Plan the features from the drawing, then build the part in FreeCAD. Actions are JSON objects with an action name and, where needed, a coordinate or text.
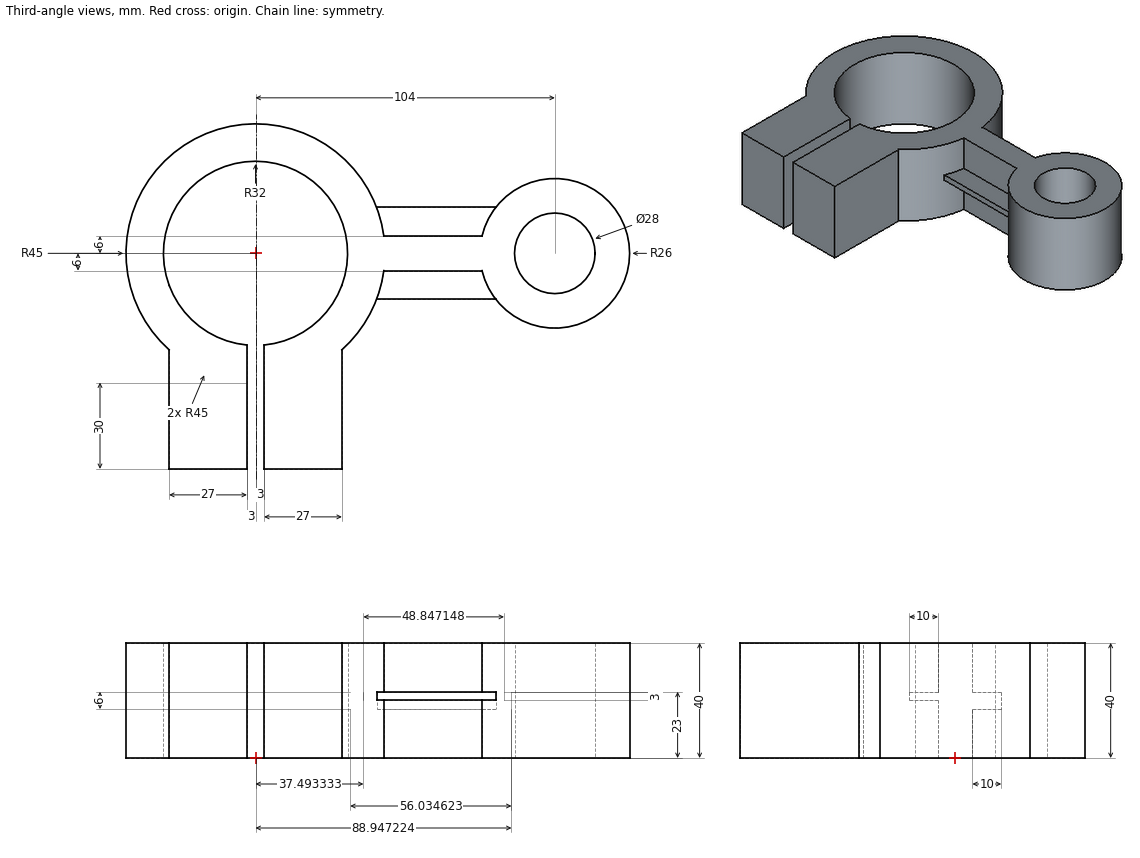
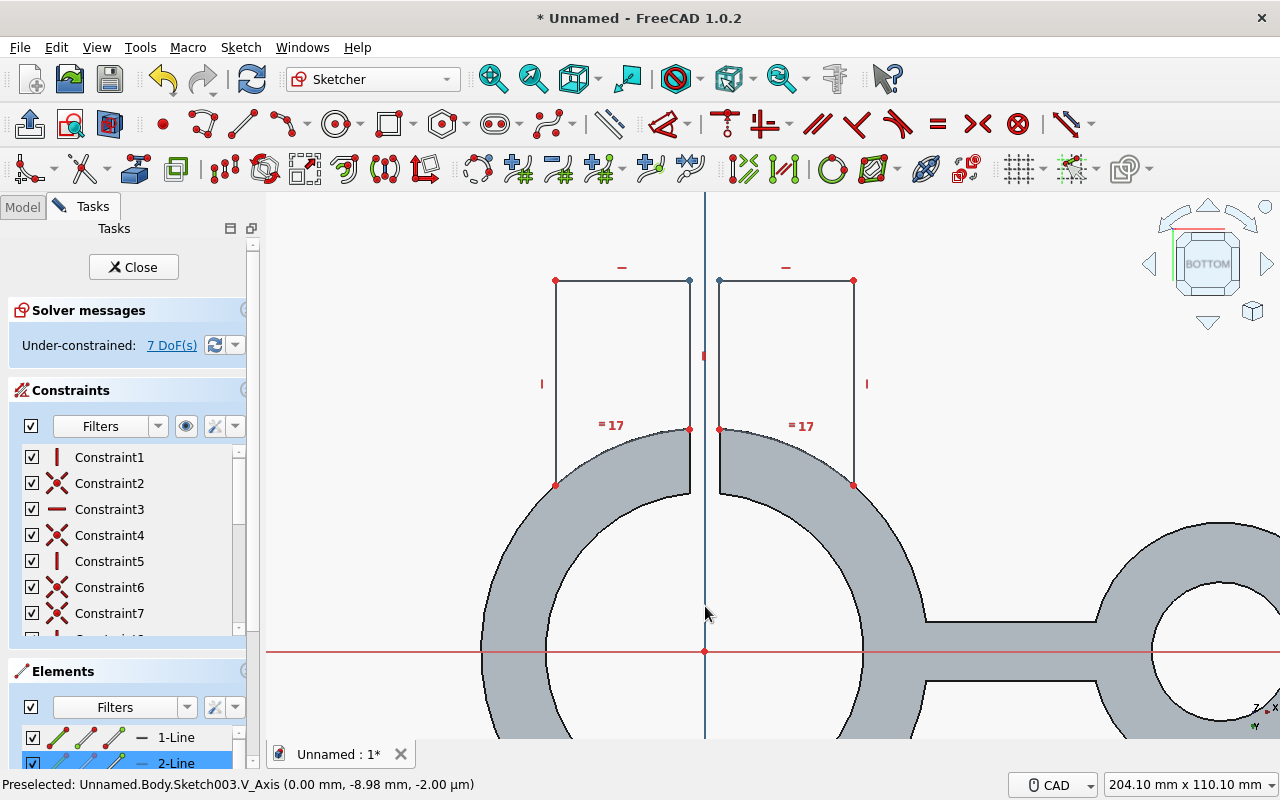
{"action": "left_click", "coordinate": [978, 124]}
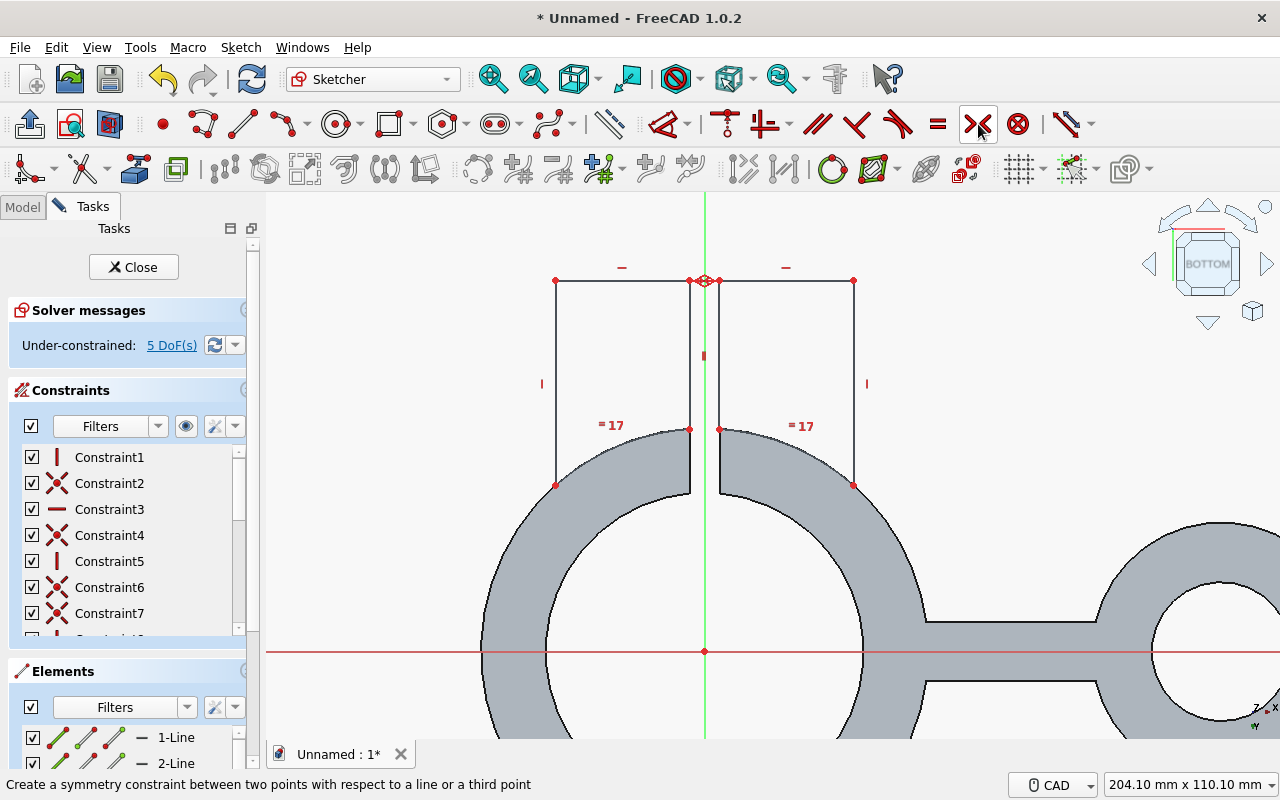
{"action": "left_click", "coordinate": [664, 124]}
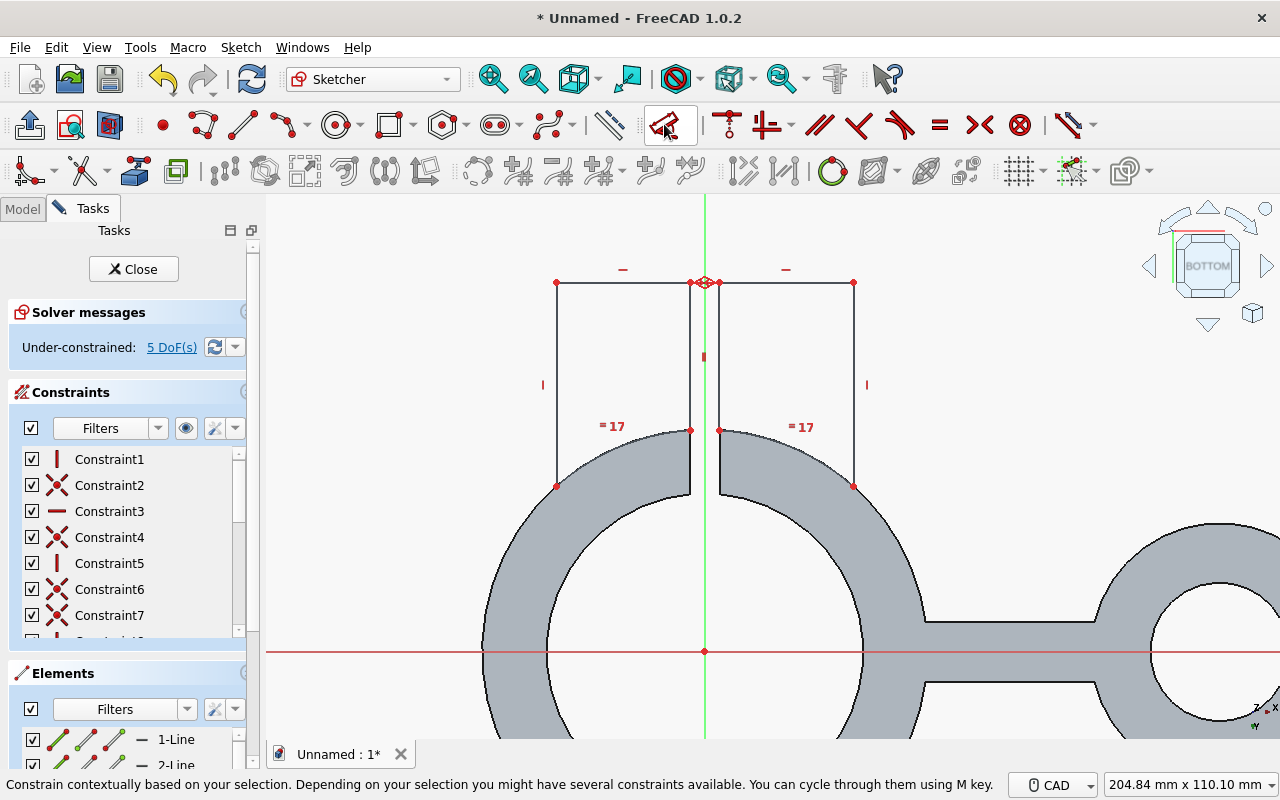
{"action": "left_click", "coordinate": [647, 437]}
{"action": "left_click", "coordinate": [639, 406]}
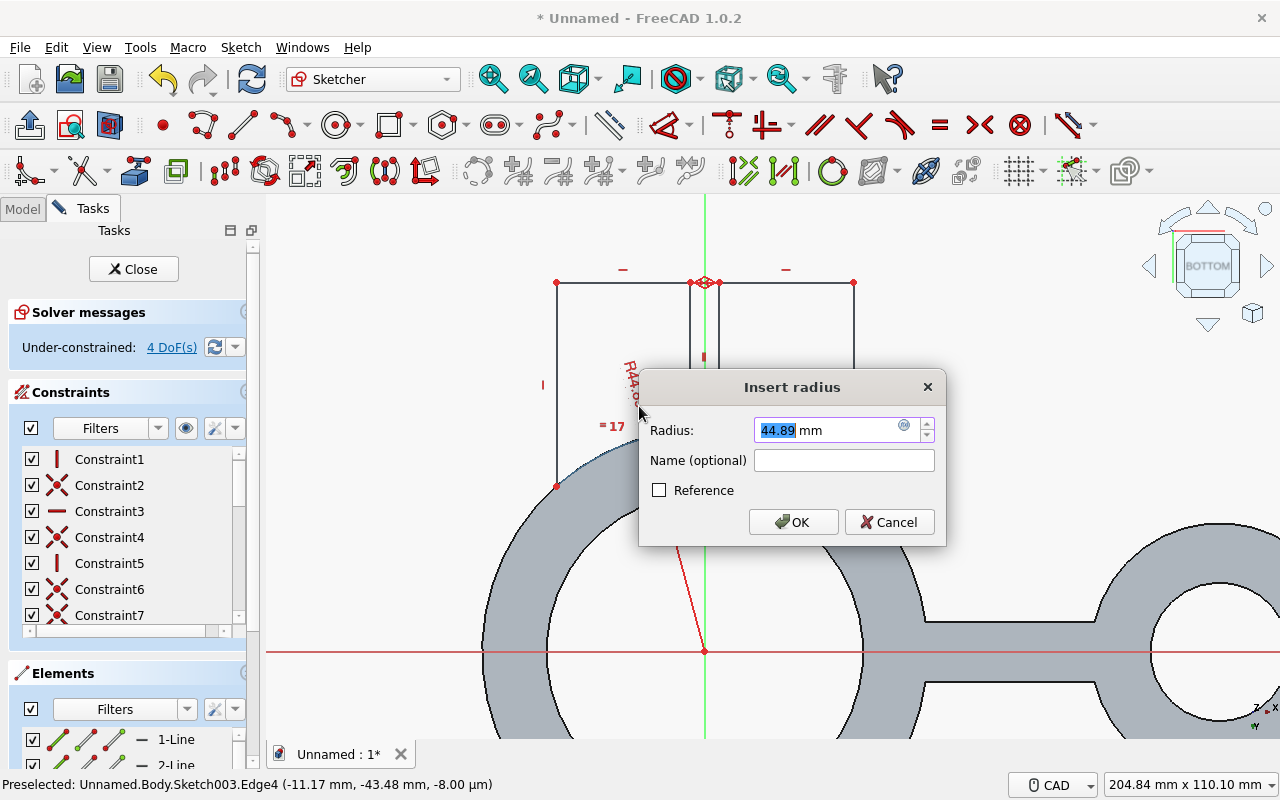
{"action": "type", "text": "45"}
{"action": "key", "text": "Return"}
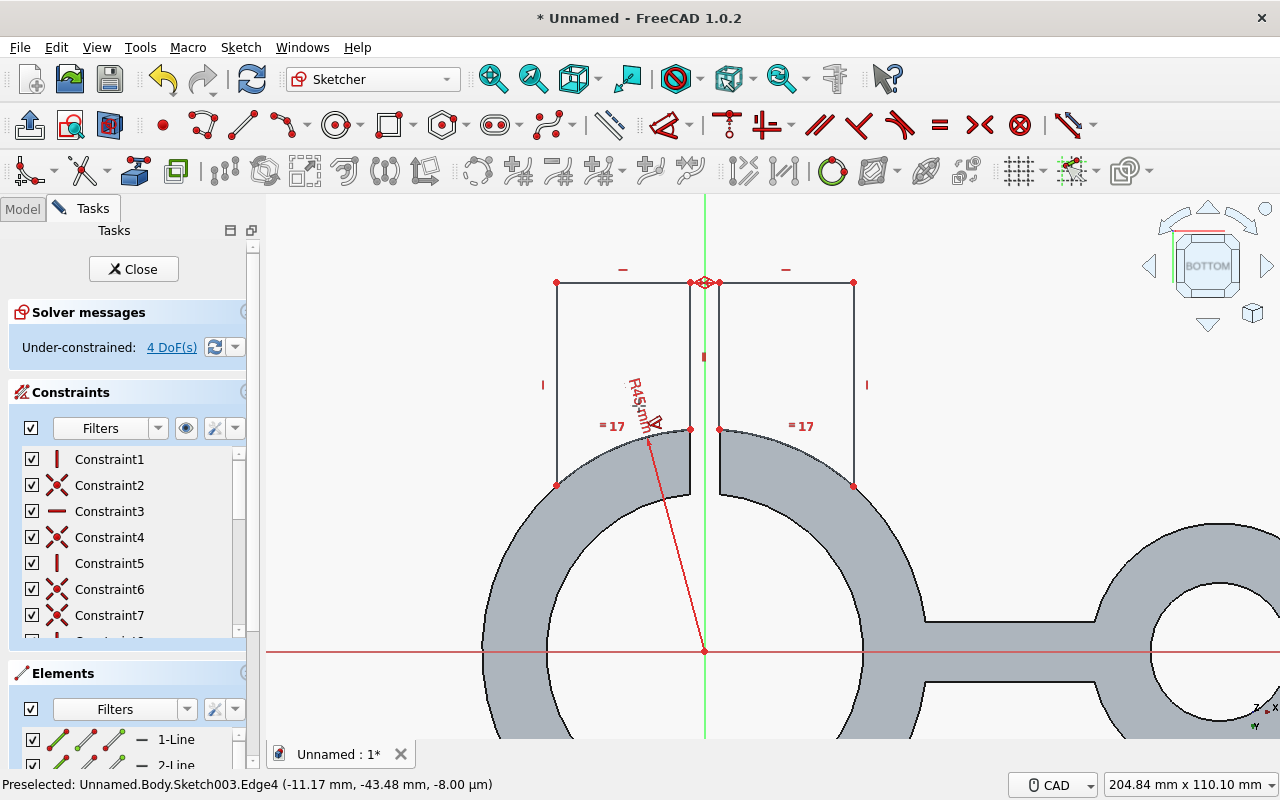
{"action": "left_click", "coordinate": [597, 283]}
{"action": "left_click", "coordinate": [624, 249]}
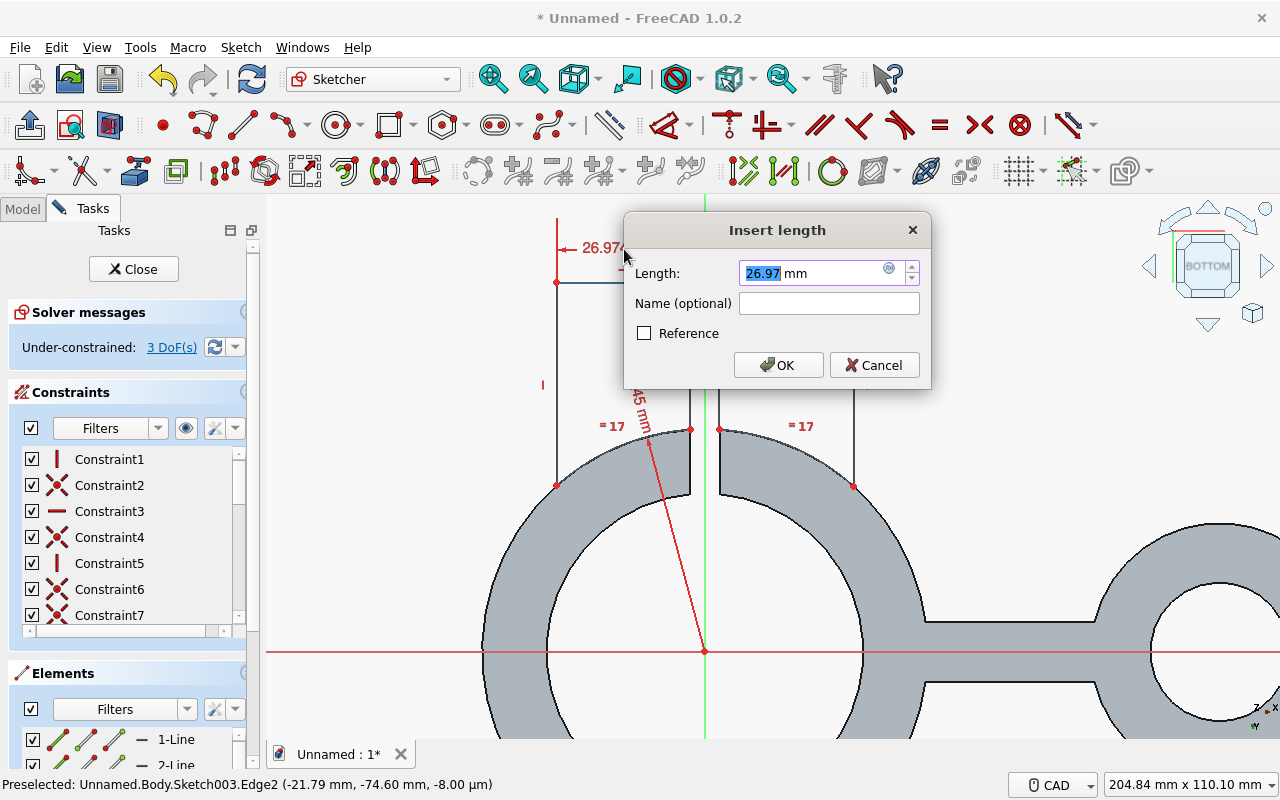
{"action": "type", "text": "27"}
{"action": "key", "text": "Return"}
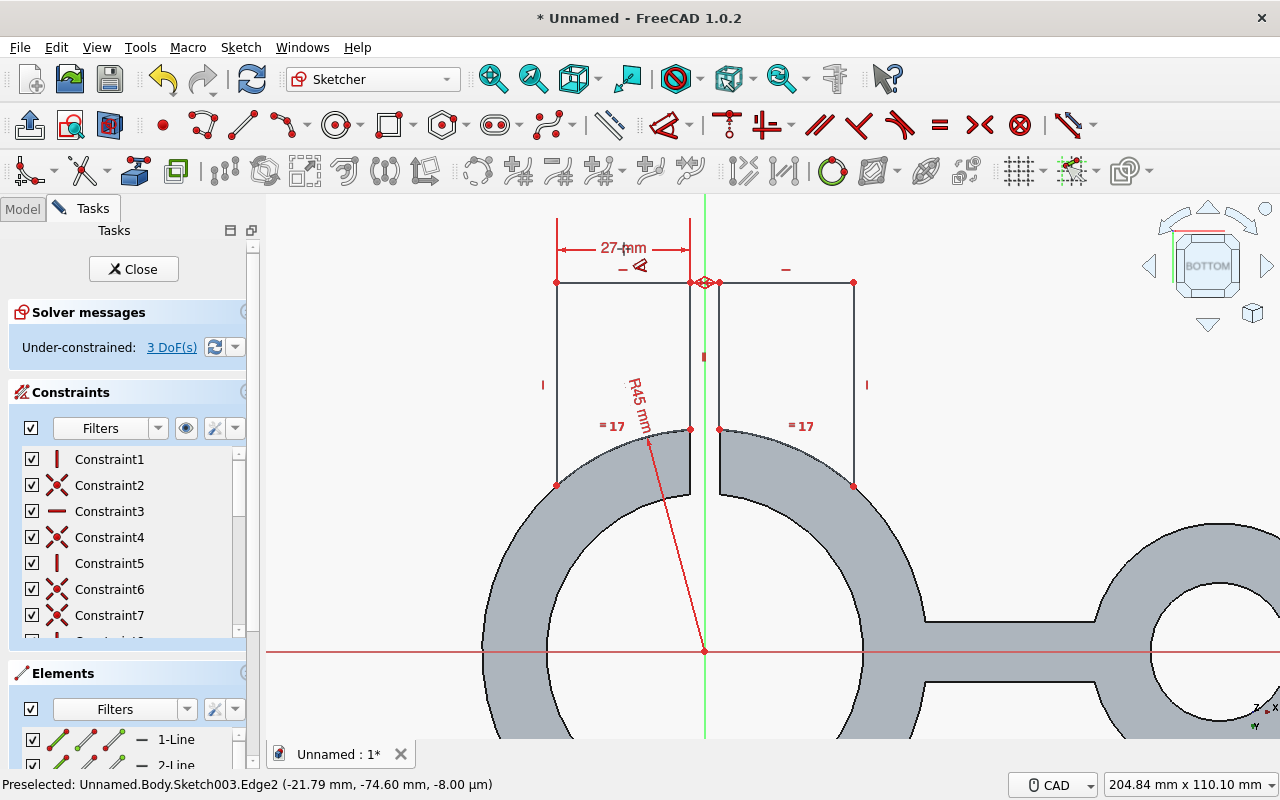
{"action": "left_click", "coordinate": [690, 327]}
{"action": "left_click", "coordinate": [656, 356]}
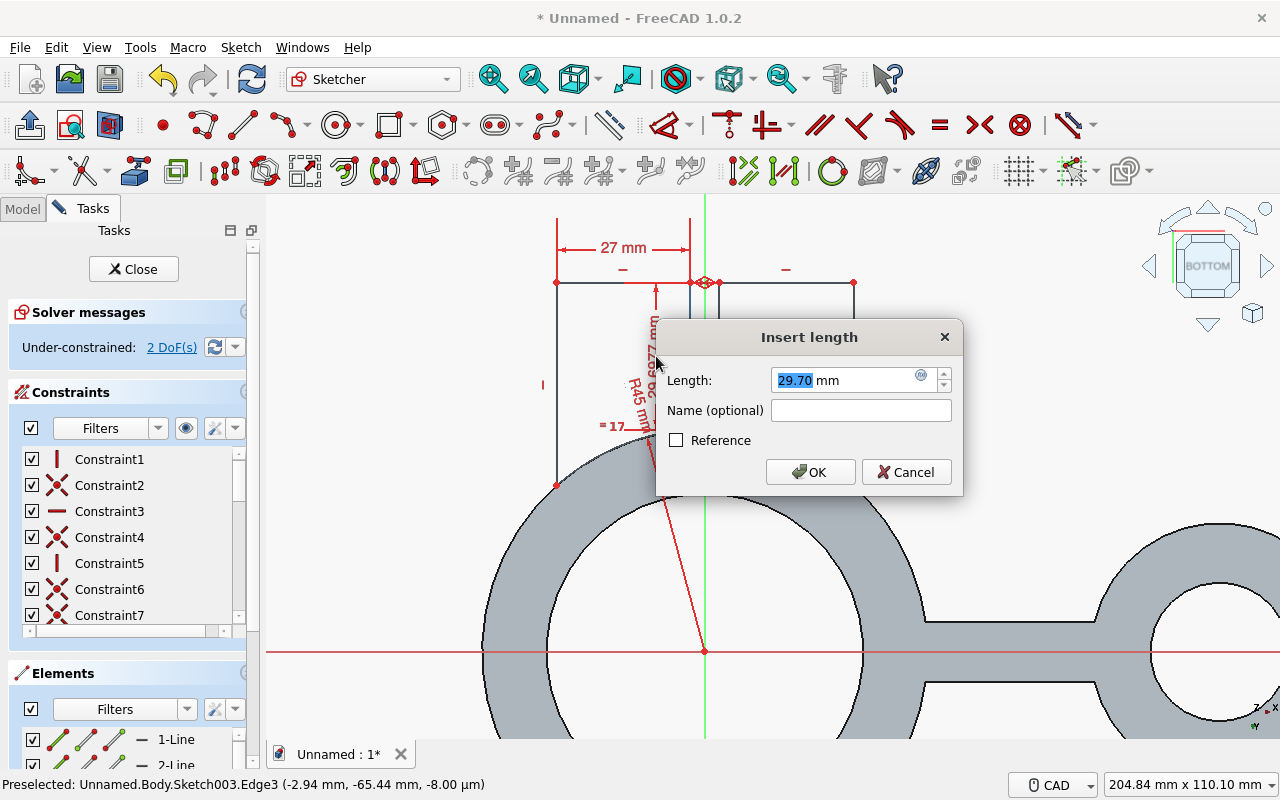
{"action": "type", "text": "30"}
{"action": "key", "text": "Return"}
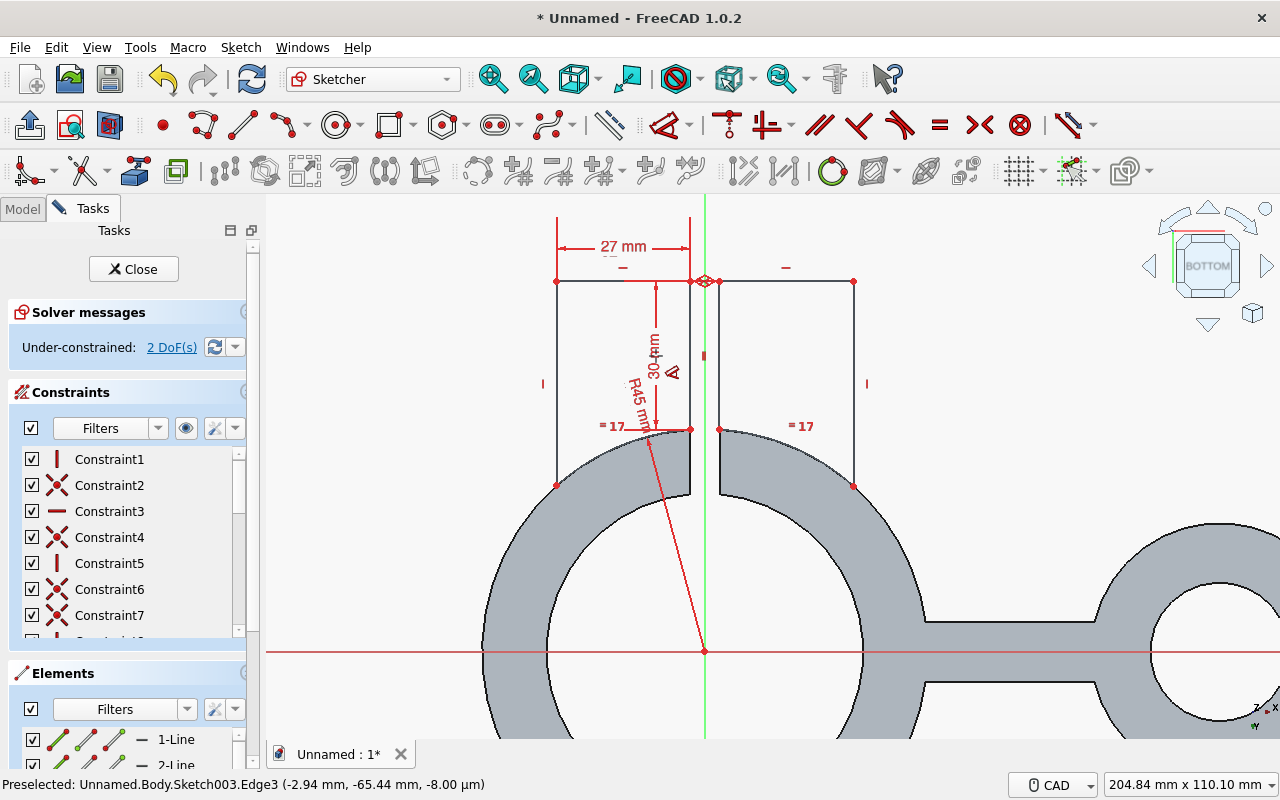
{"action": "left_click", "coordinate": [760, 281]}
{"action": "left_click", "coordinate": [787, 247]}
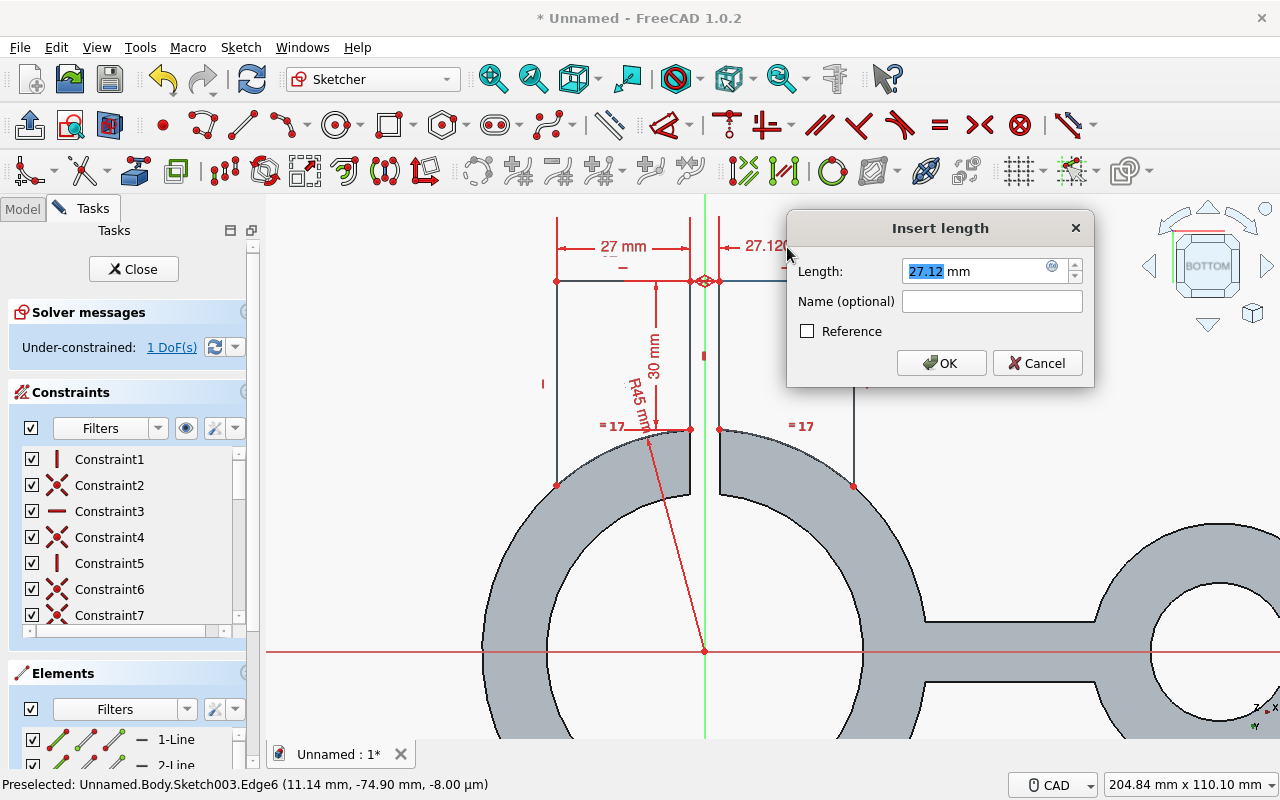
{"action": "type", "text": "27"}
{"action": "key", "text": "Return"}